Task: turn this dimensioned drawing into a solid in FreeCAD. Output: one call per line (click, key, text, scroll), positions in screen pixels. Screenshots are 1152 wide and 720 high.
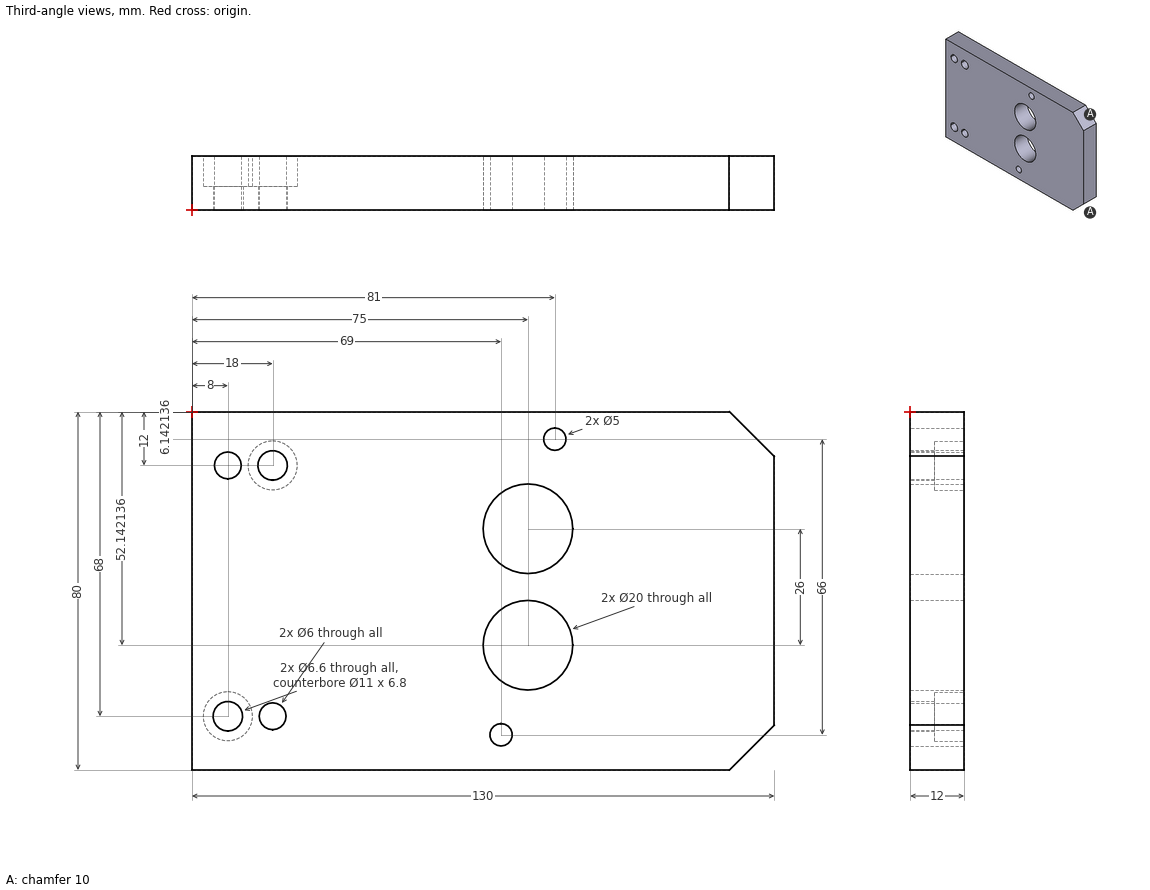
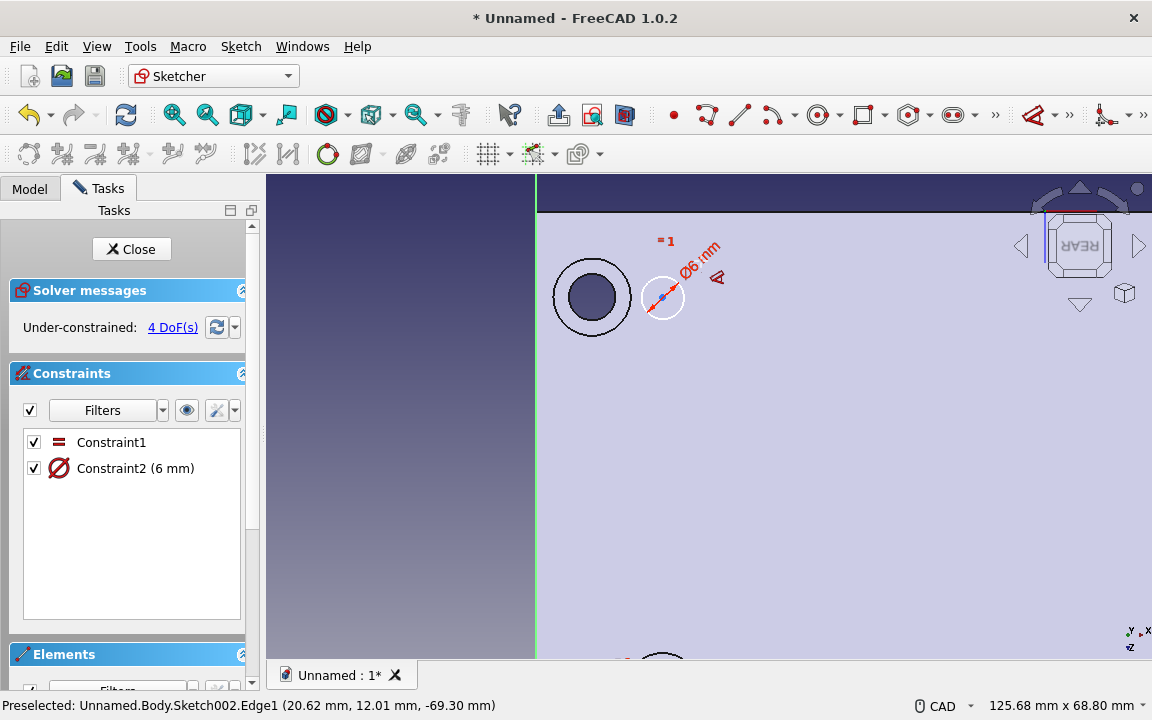
scroll(678, 283, down, 3)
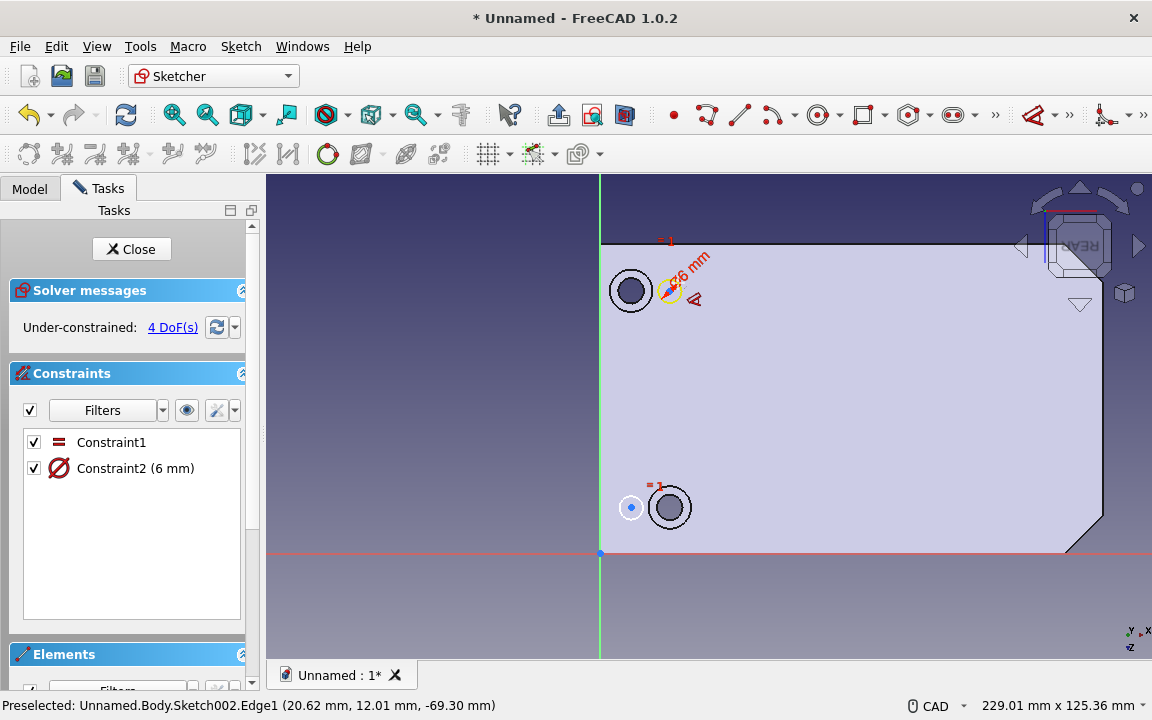
scroll(631, 508, up, 2)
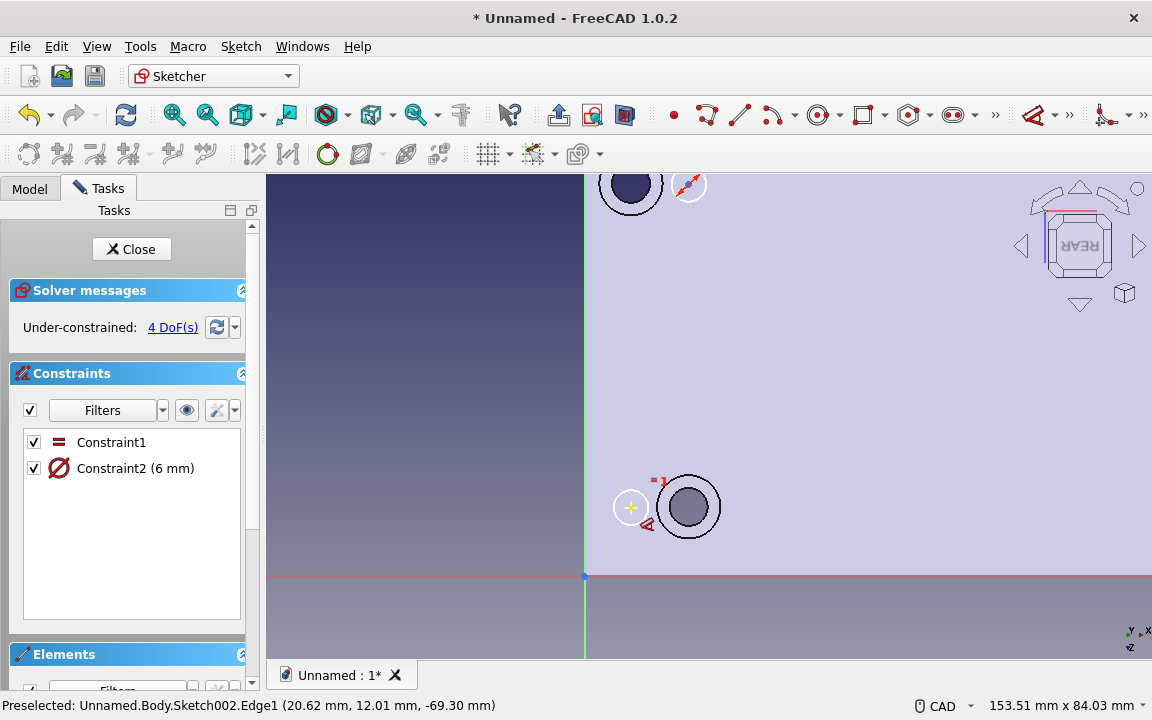
click(631, 508)
click(608, 610)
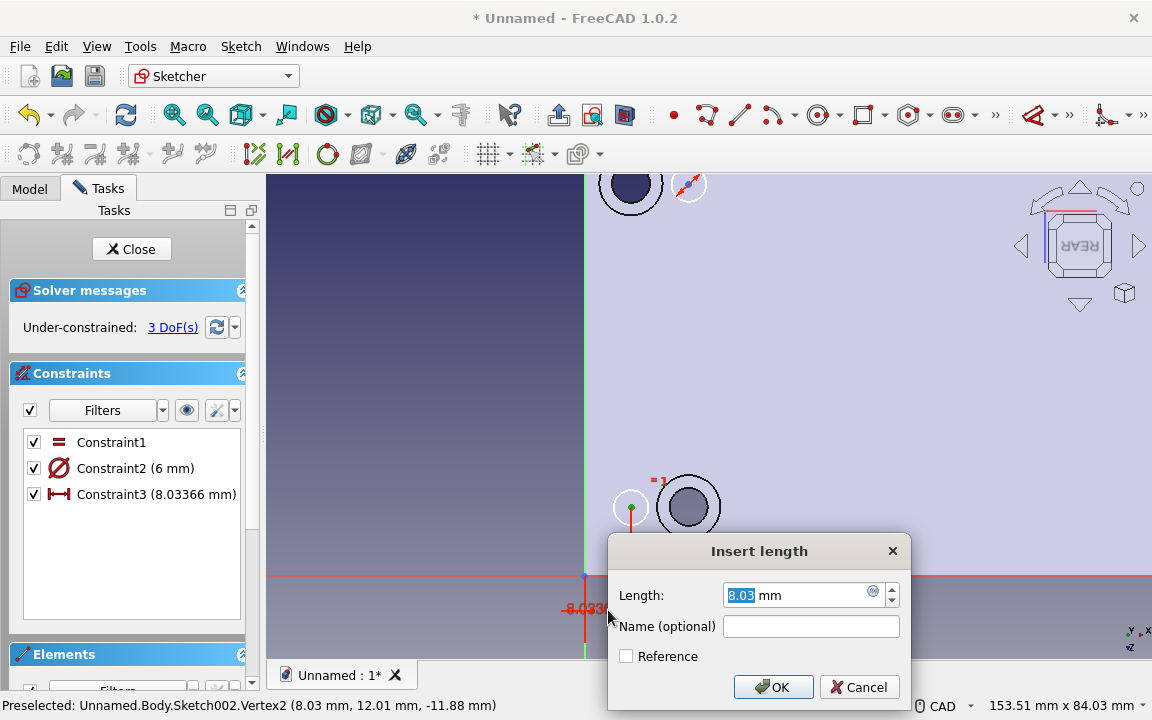
text(8)
key(Return)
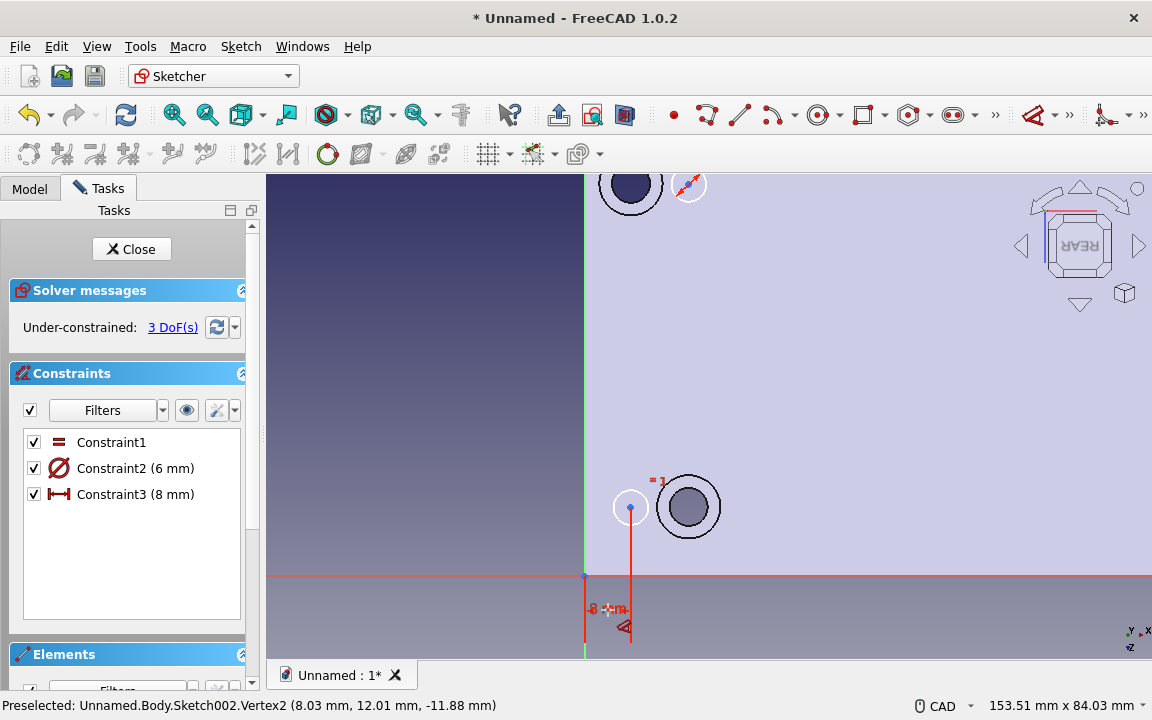
scroll(631, 509, down, 2)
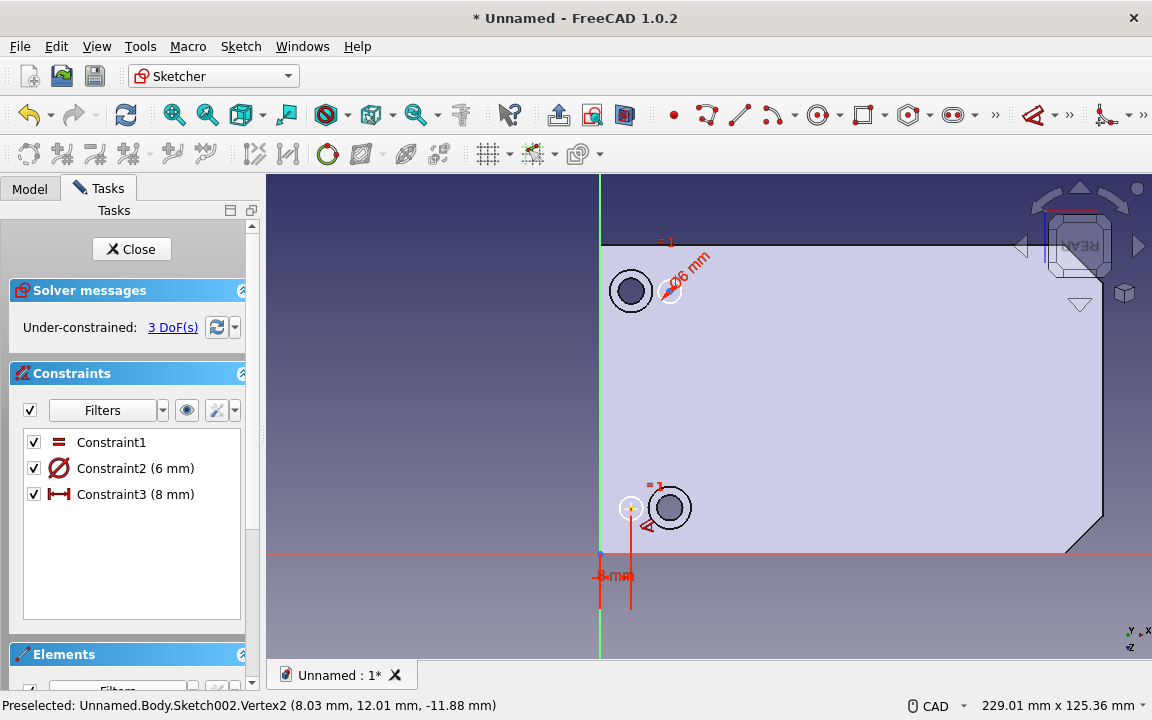
click(670, 292)
click(619, 258)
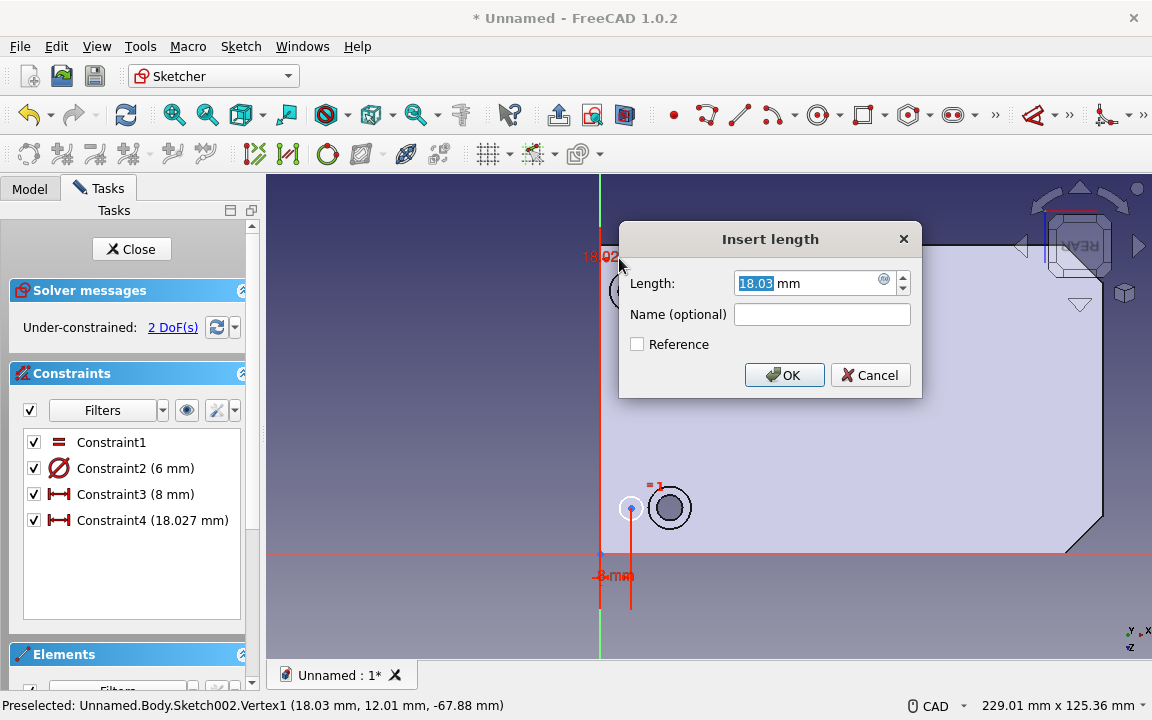
text(18)
key(Return)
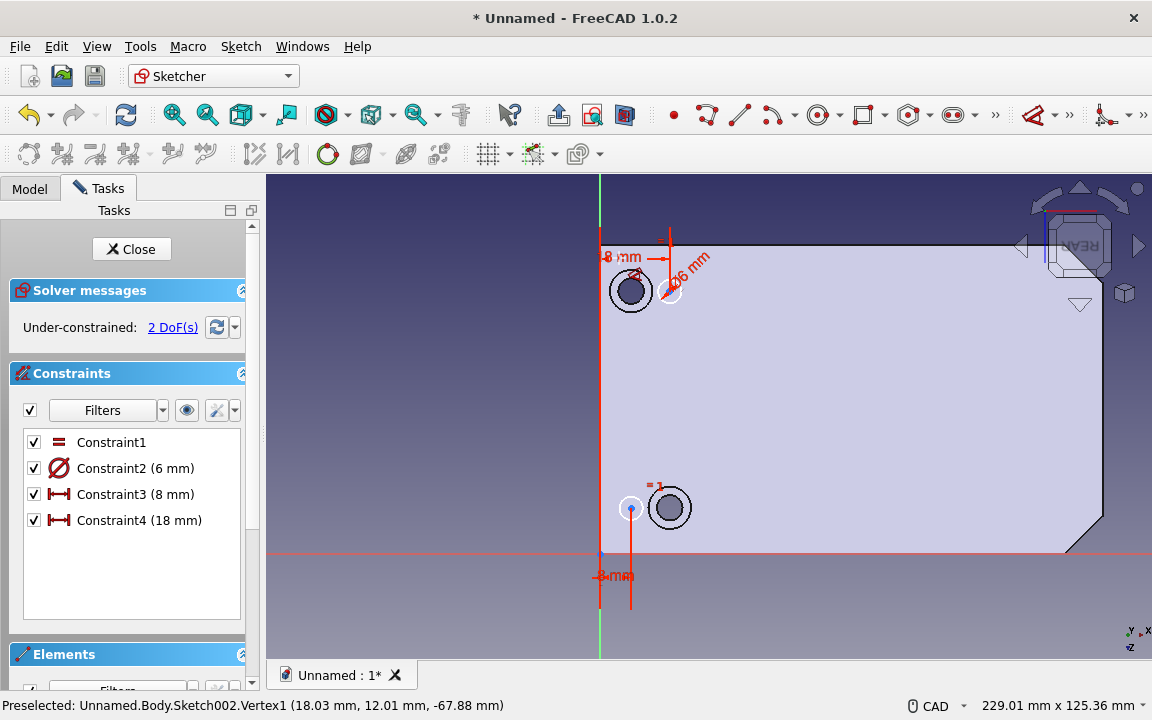
click(670, 292)
click(566, 423)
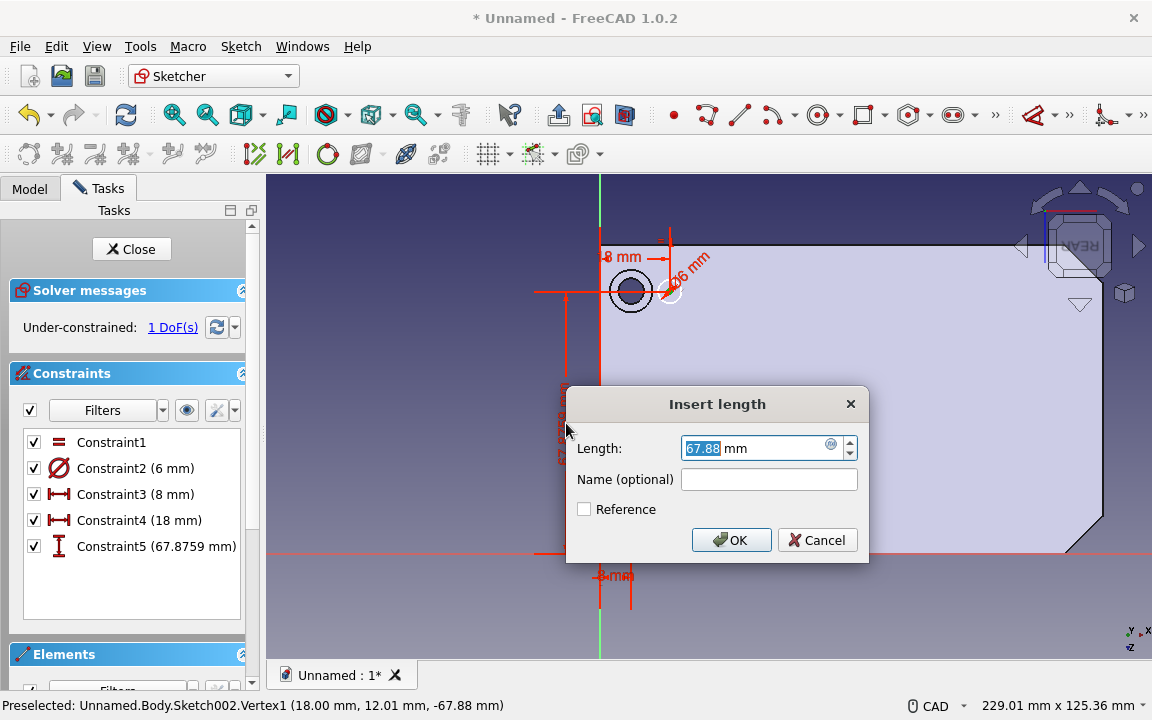
text(68)
key(Return)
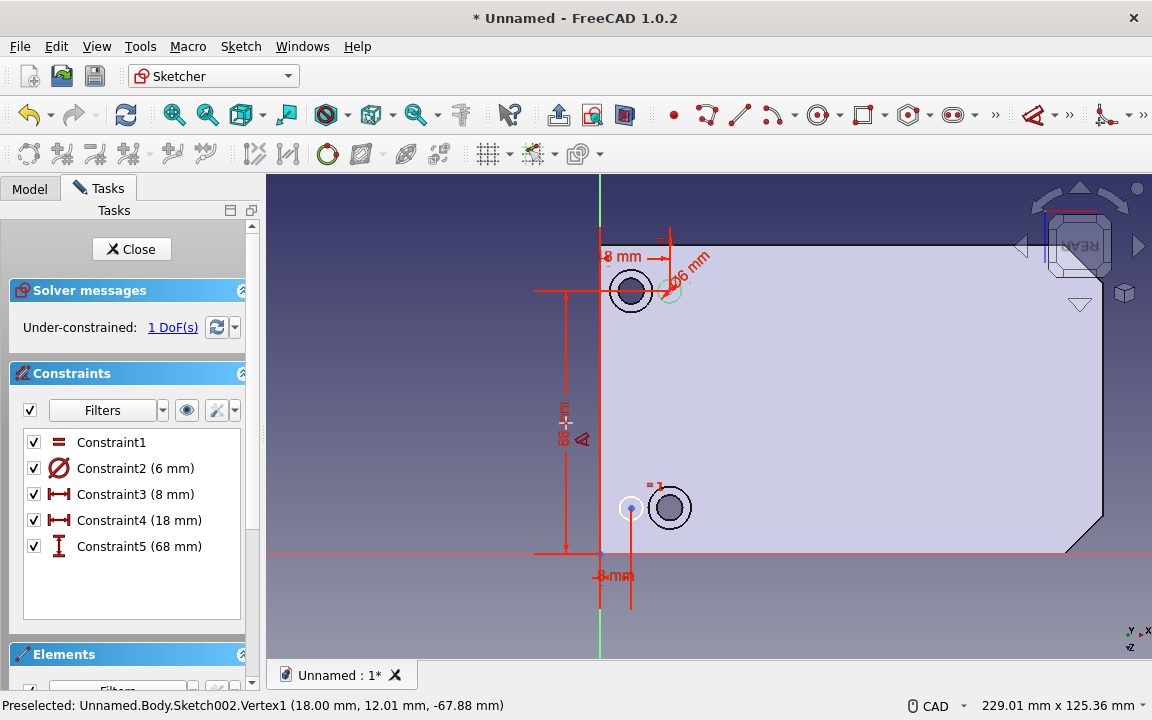
click(631, 508)
click(566, 531)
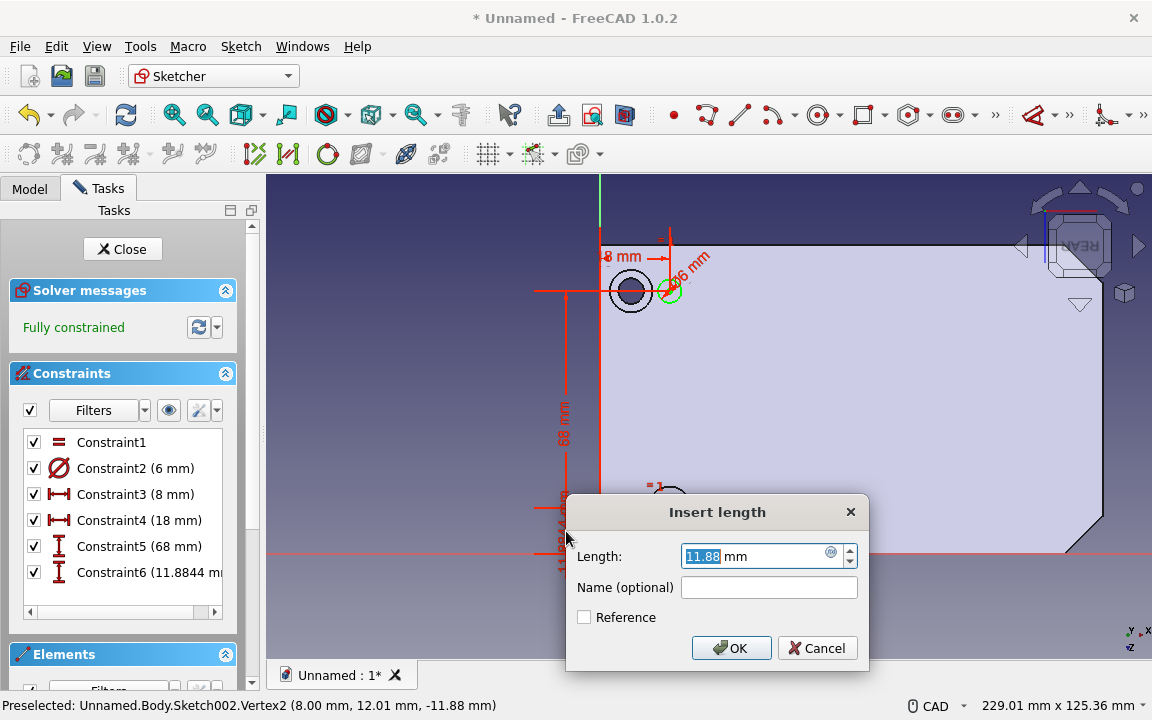
text(12)
key(Return)
key(Escape)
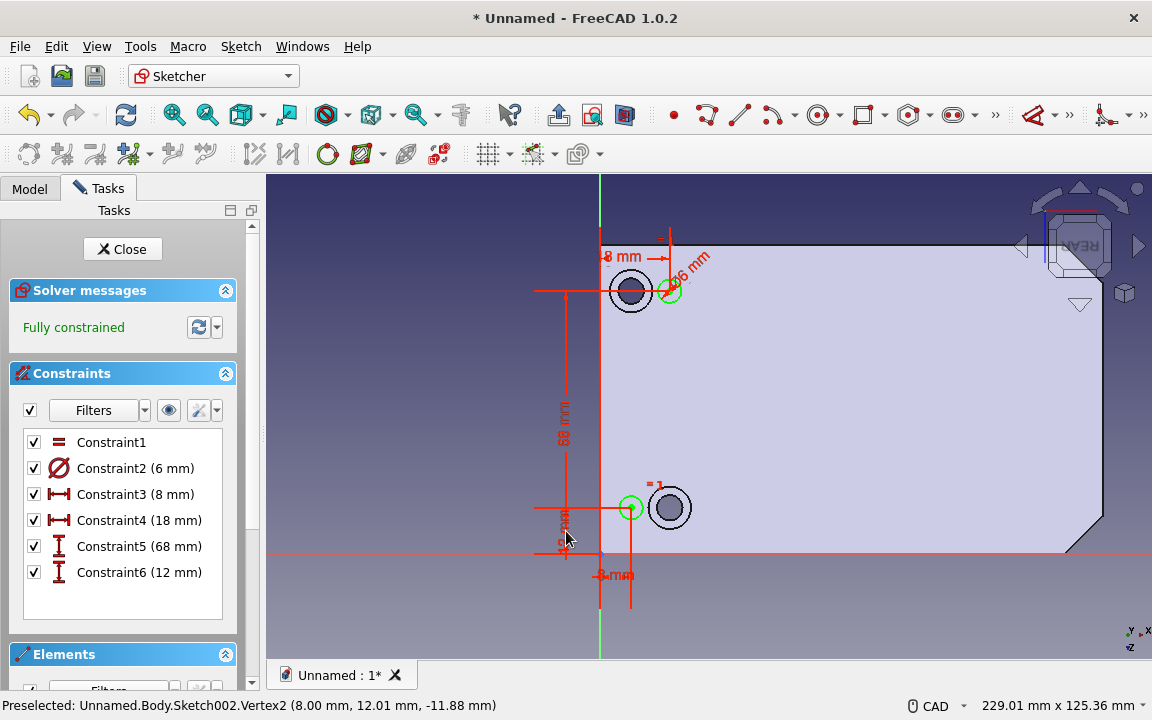
click(123, 249)